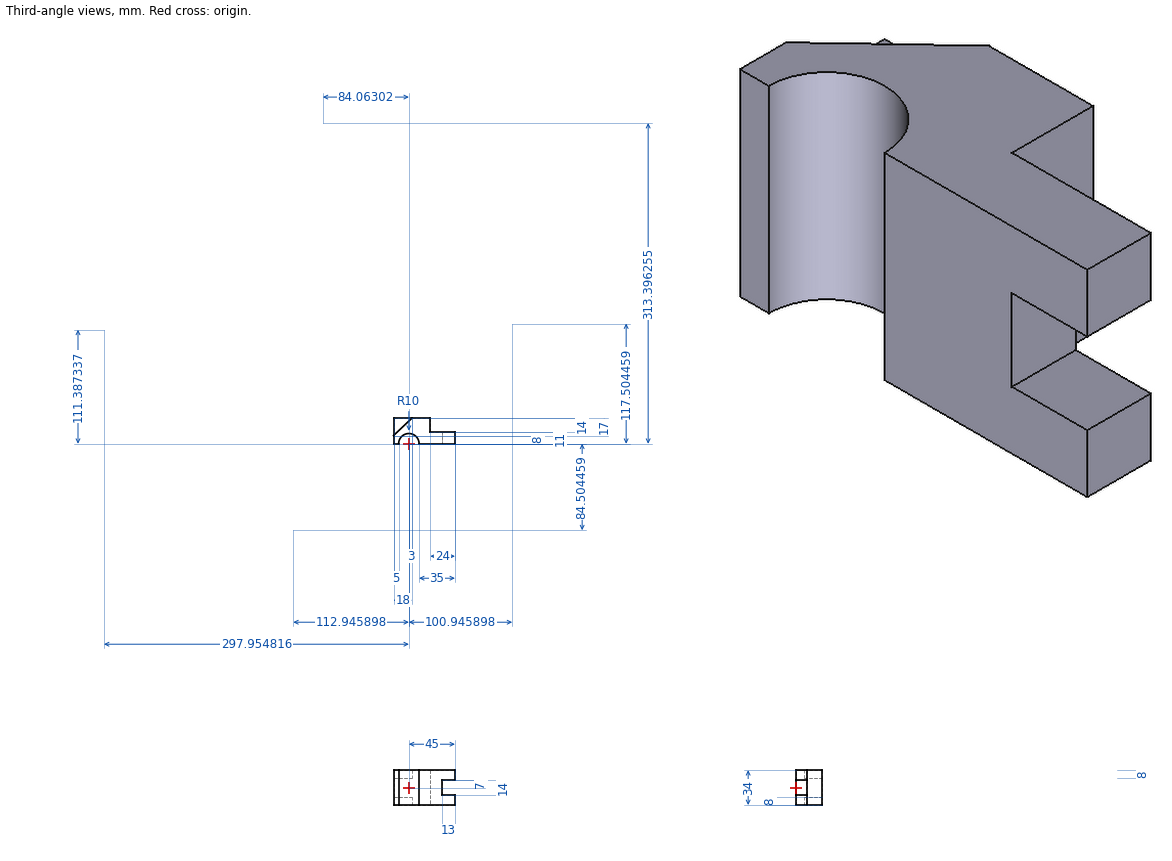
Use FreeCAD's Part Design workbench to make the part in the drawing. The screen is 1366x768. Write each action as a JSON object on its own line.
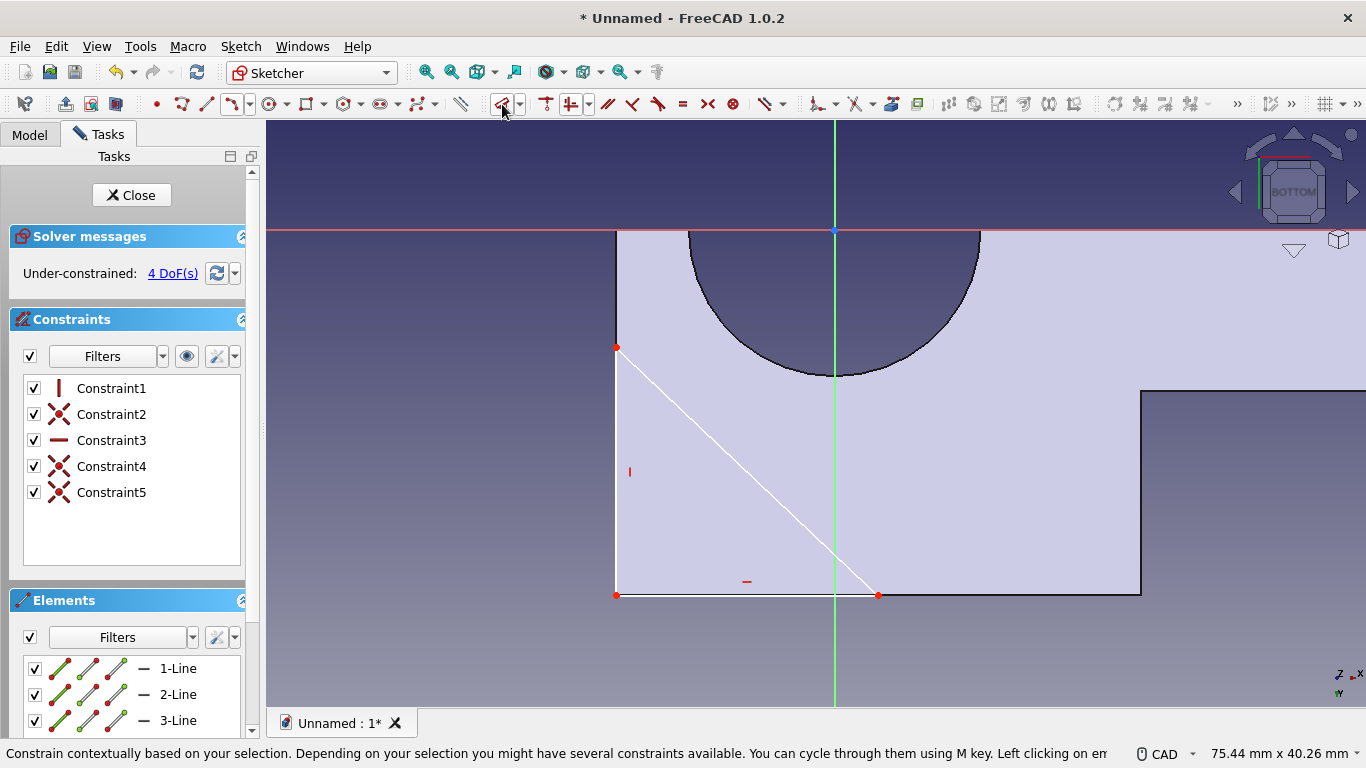
{"action": "left_click", "coordinate": [616, 422]}
{"action": "left_click", "coordinate": [582, 472]}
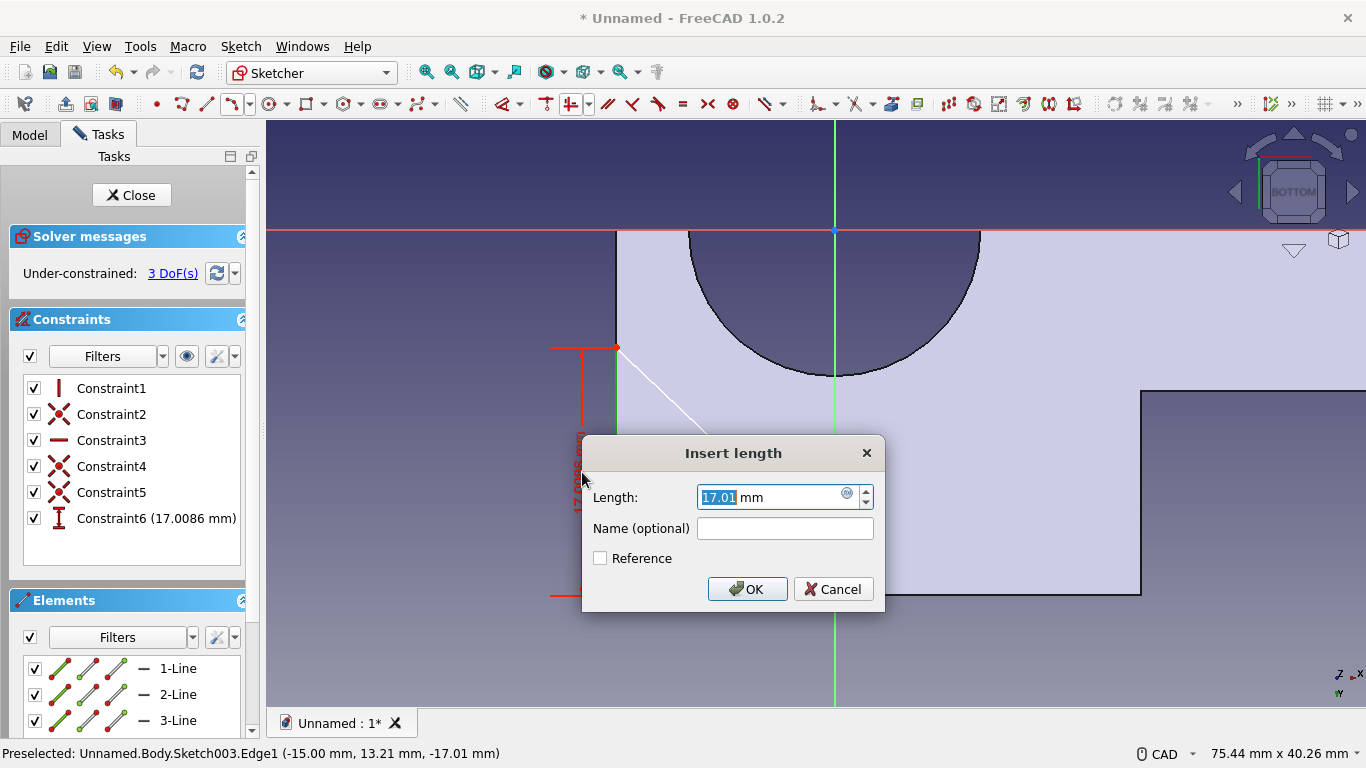
{"action": "type", "text": "17"}
{"action": "key", "text": "Return"}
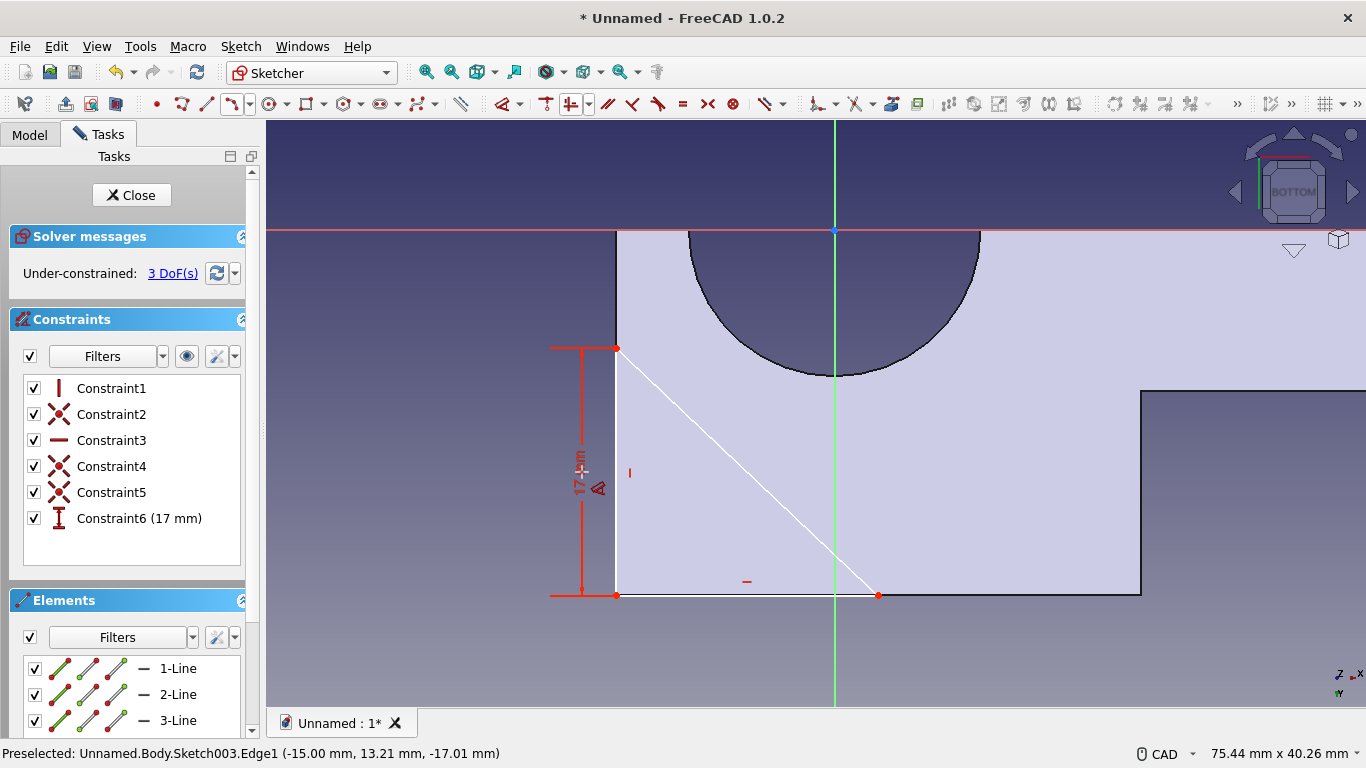
{"action": "left_click", "coordinate": [695, 596]}
{"action": "left_click", "coordinate": [747, 630]}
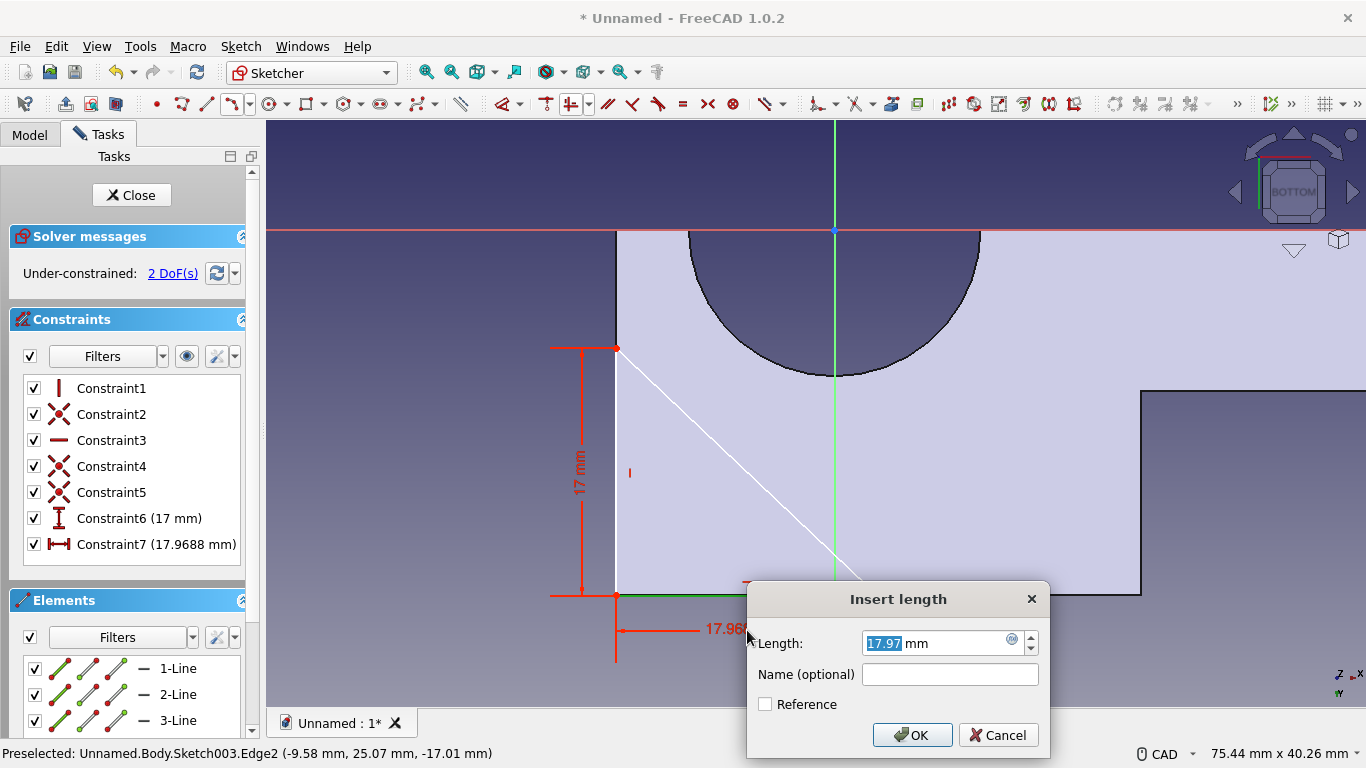
{"action": "type", "text": "18"}
{"action": "key", "text": "Return"}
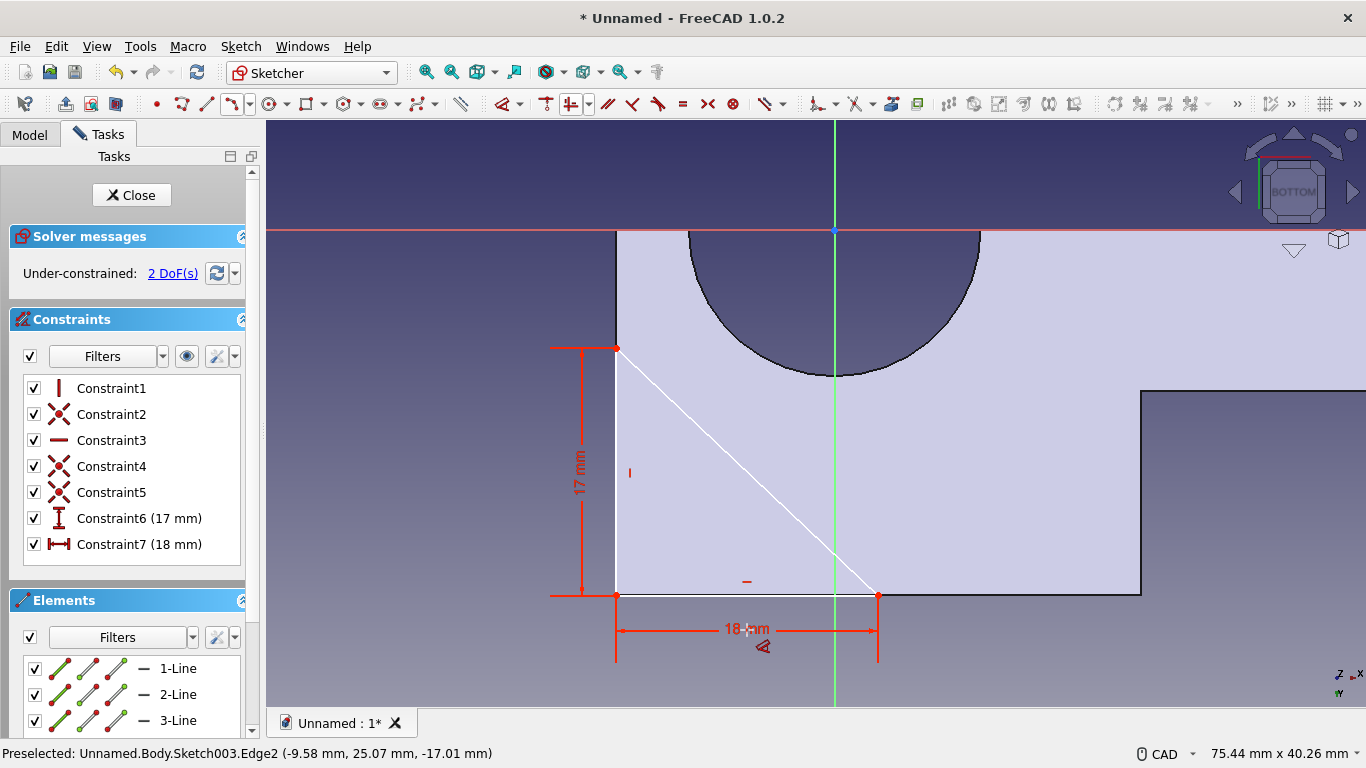
{"action": "left_click", "coordinate": [616, 348]}
{"action": "left_click", "coordinate": [582, 289]}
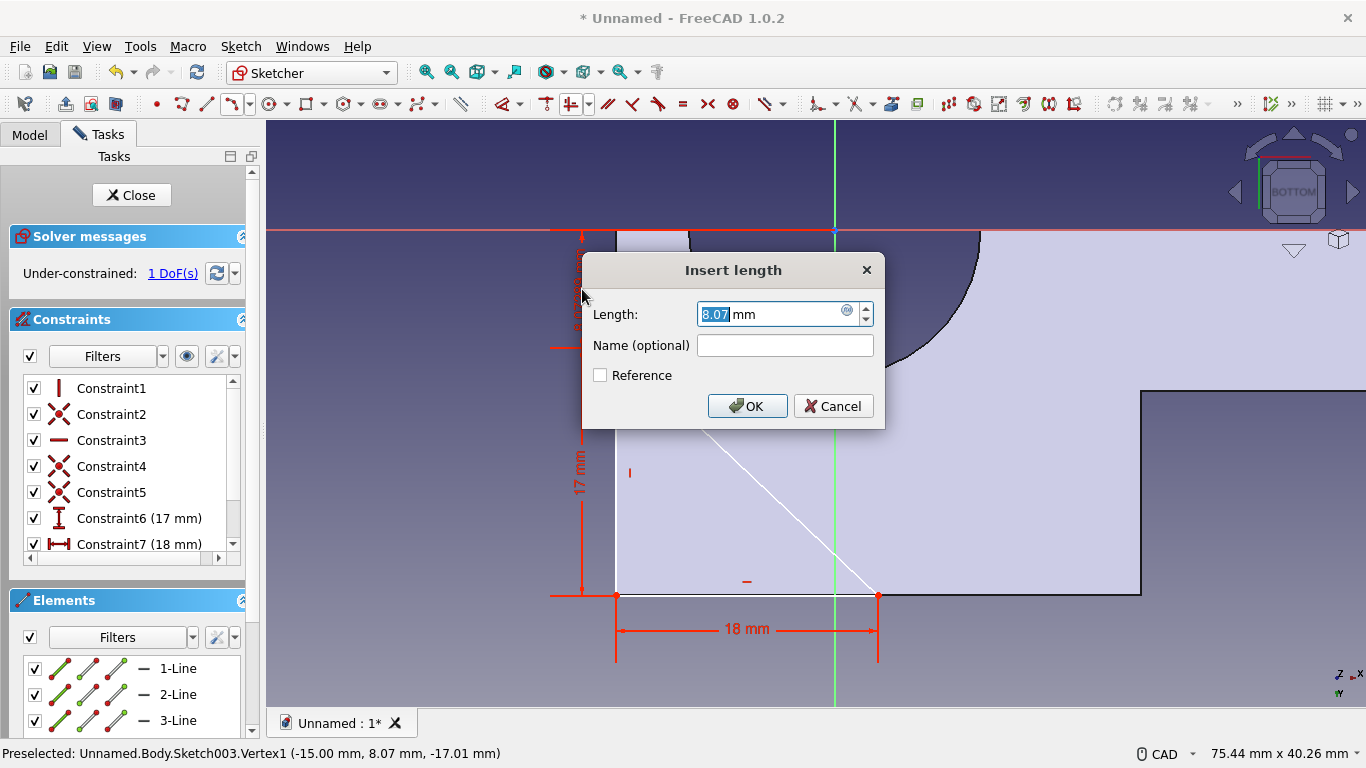
{"action": "type", "text": "8"}
{"action": "key", "text": "Return"}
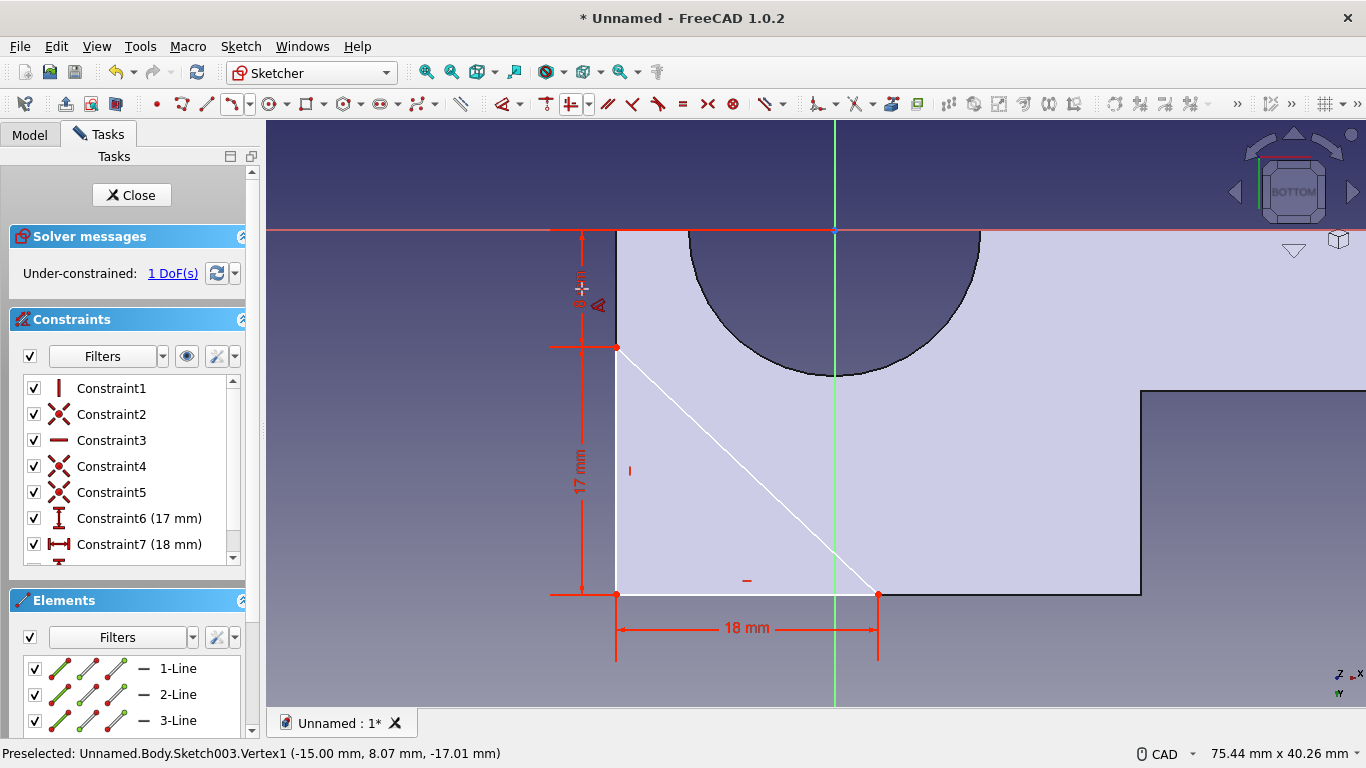
{"action": "left_click", "coordinate": [878, 595]}
{"action": "left_click", "coordinate": [857, 629]}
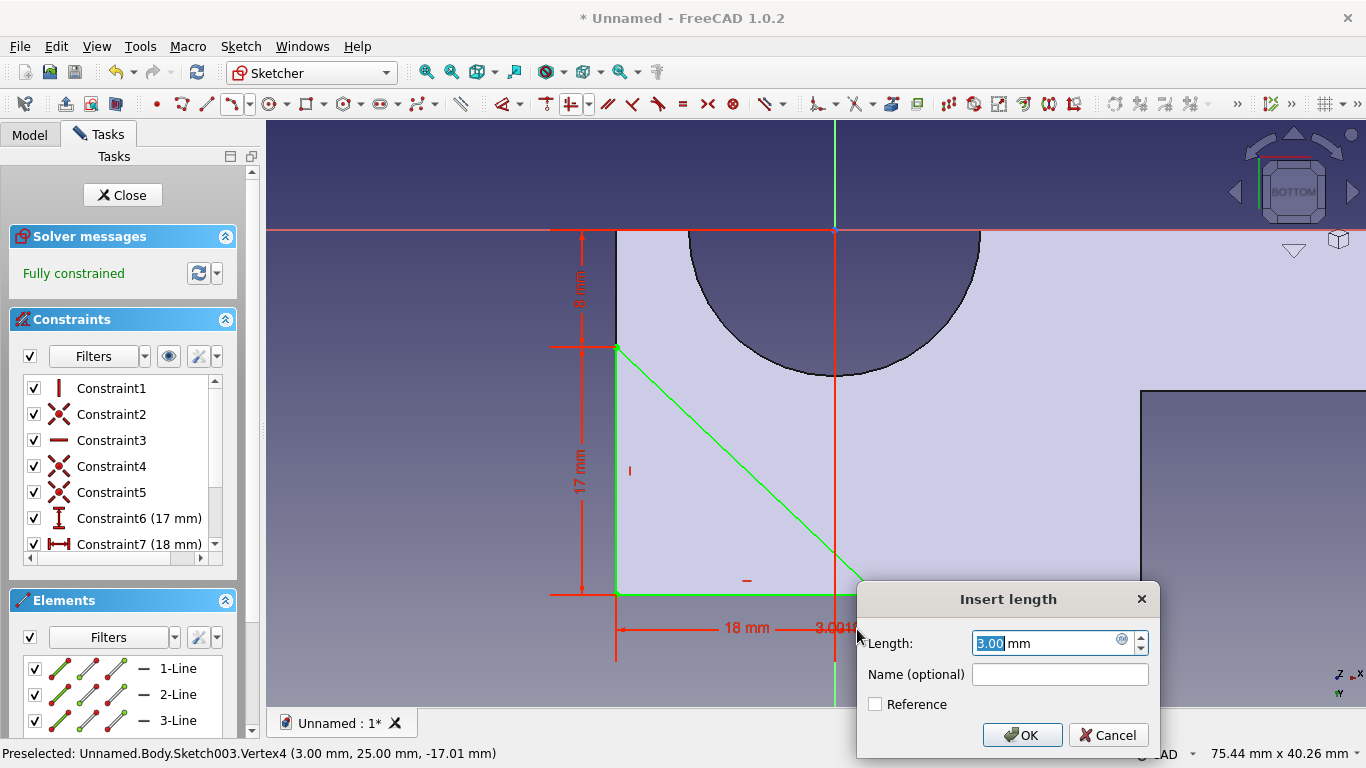
{"action": "type", "text": "3"}
{"action": "key", "text": "Return"}
{"action": "key", "text": "Escape"}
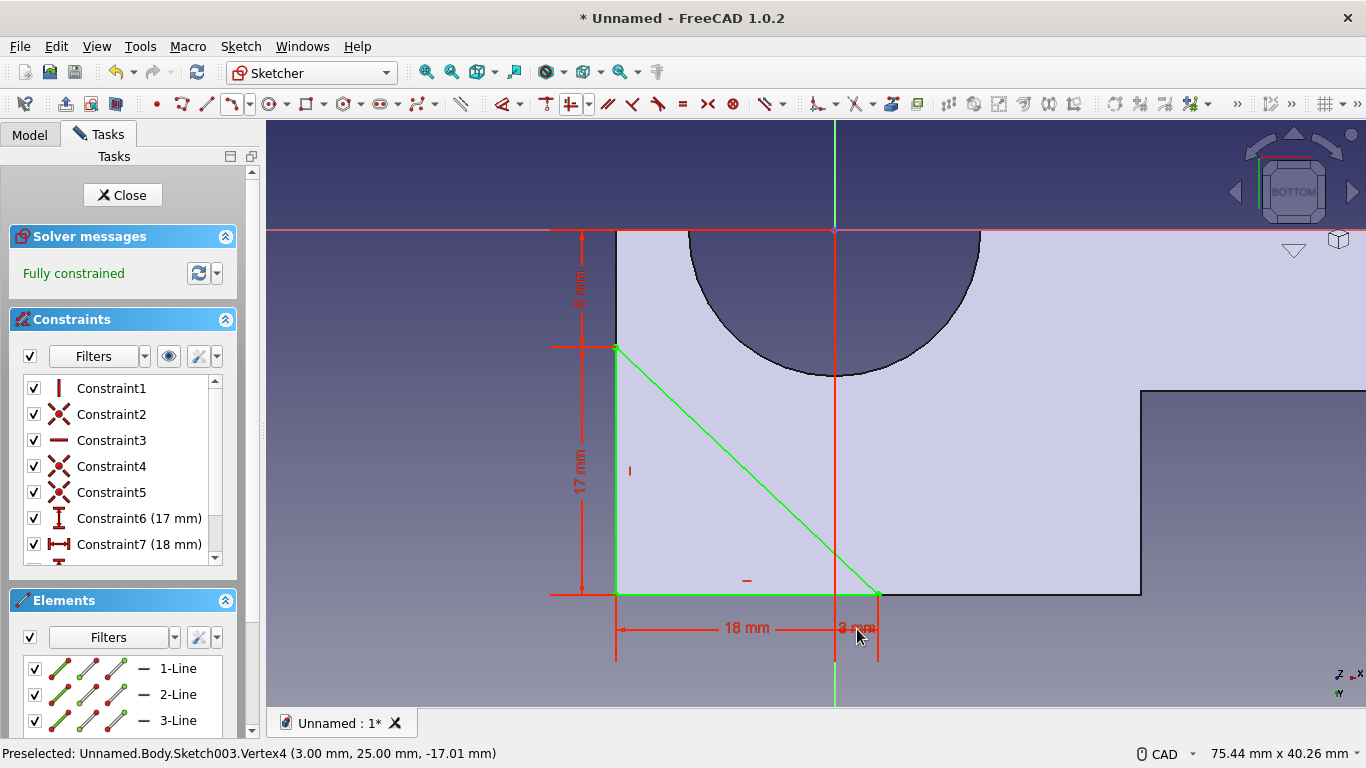
{"action": "left_click", "coordinate": [123, 195]}